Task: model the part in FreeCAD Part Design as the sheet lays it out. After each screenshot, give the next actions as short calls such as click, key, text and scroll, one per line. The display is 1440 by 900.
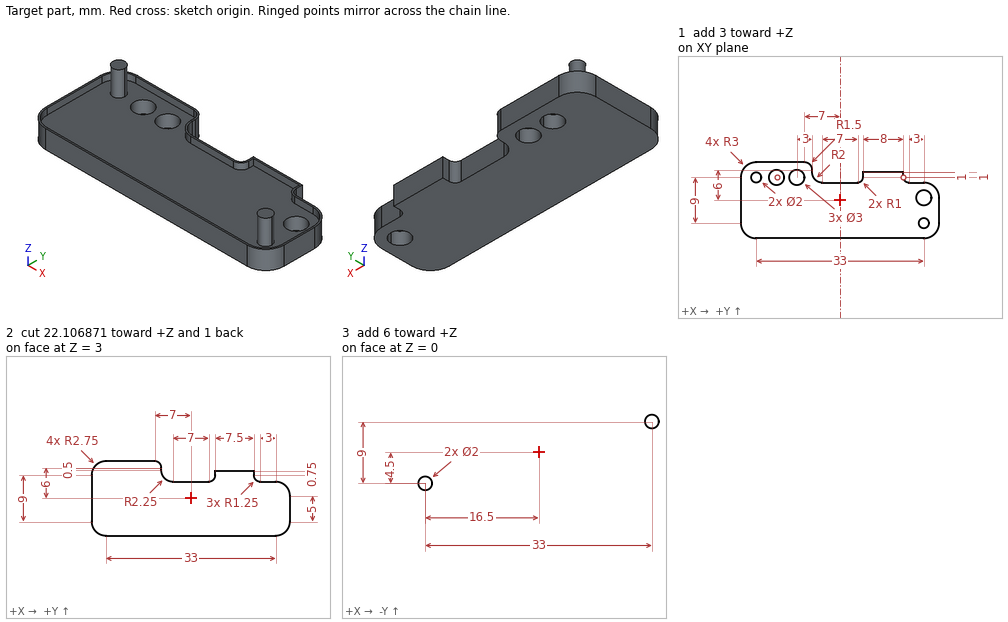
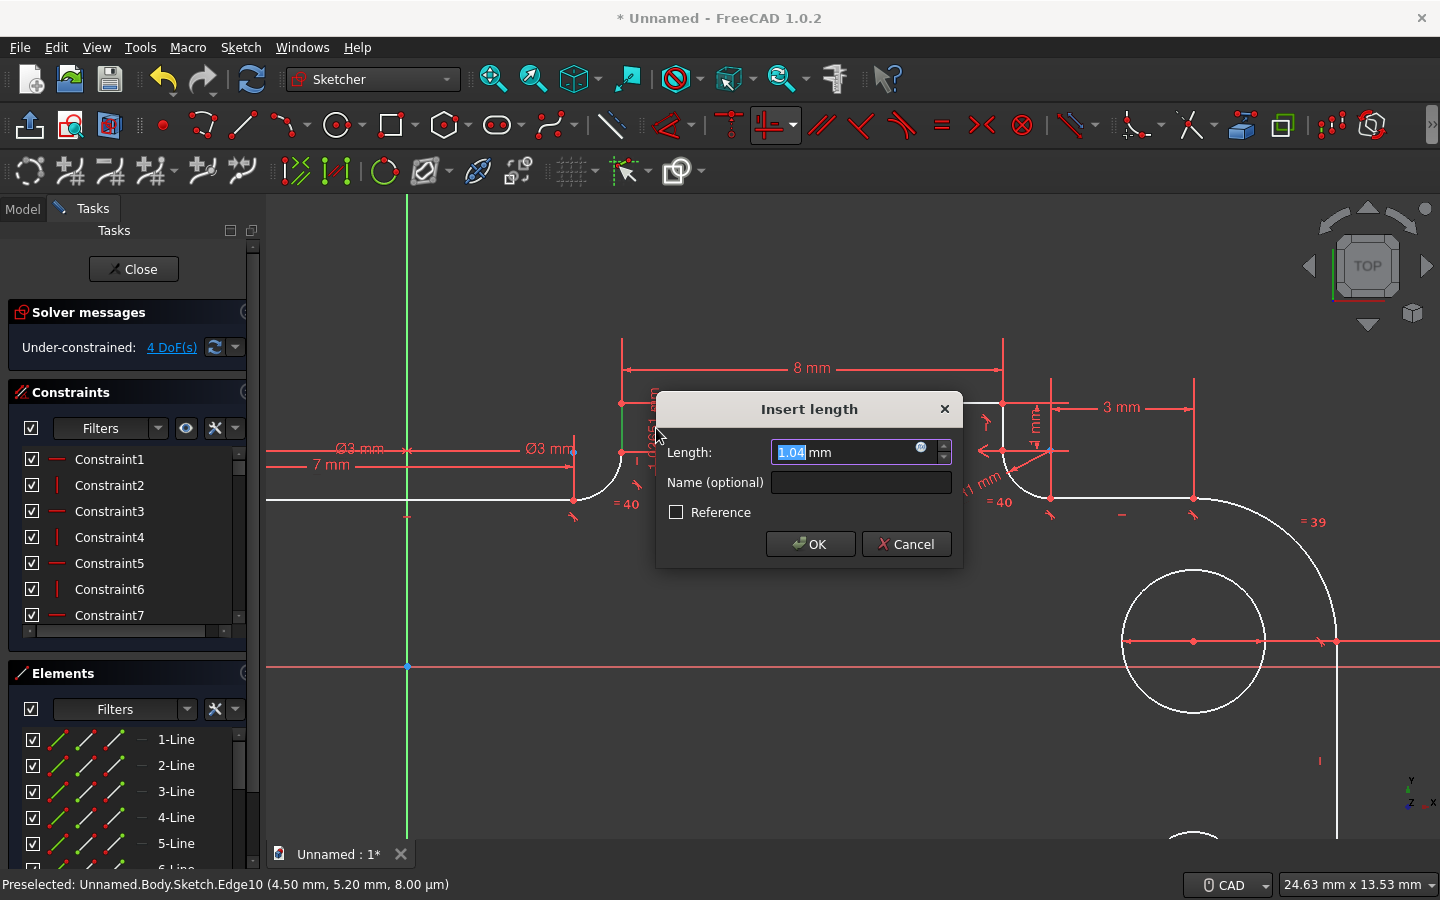
text(1)
key(Return)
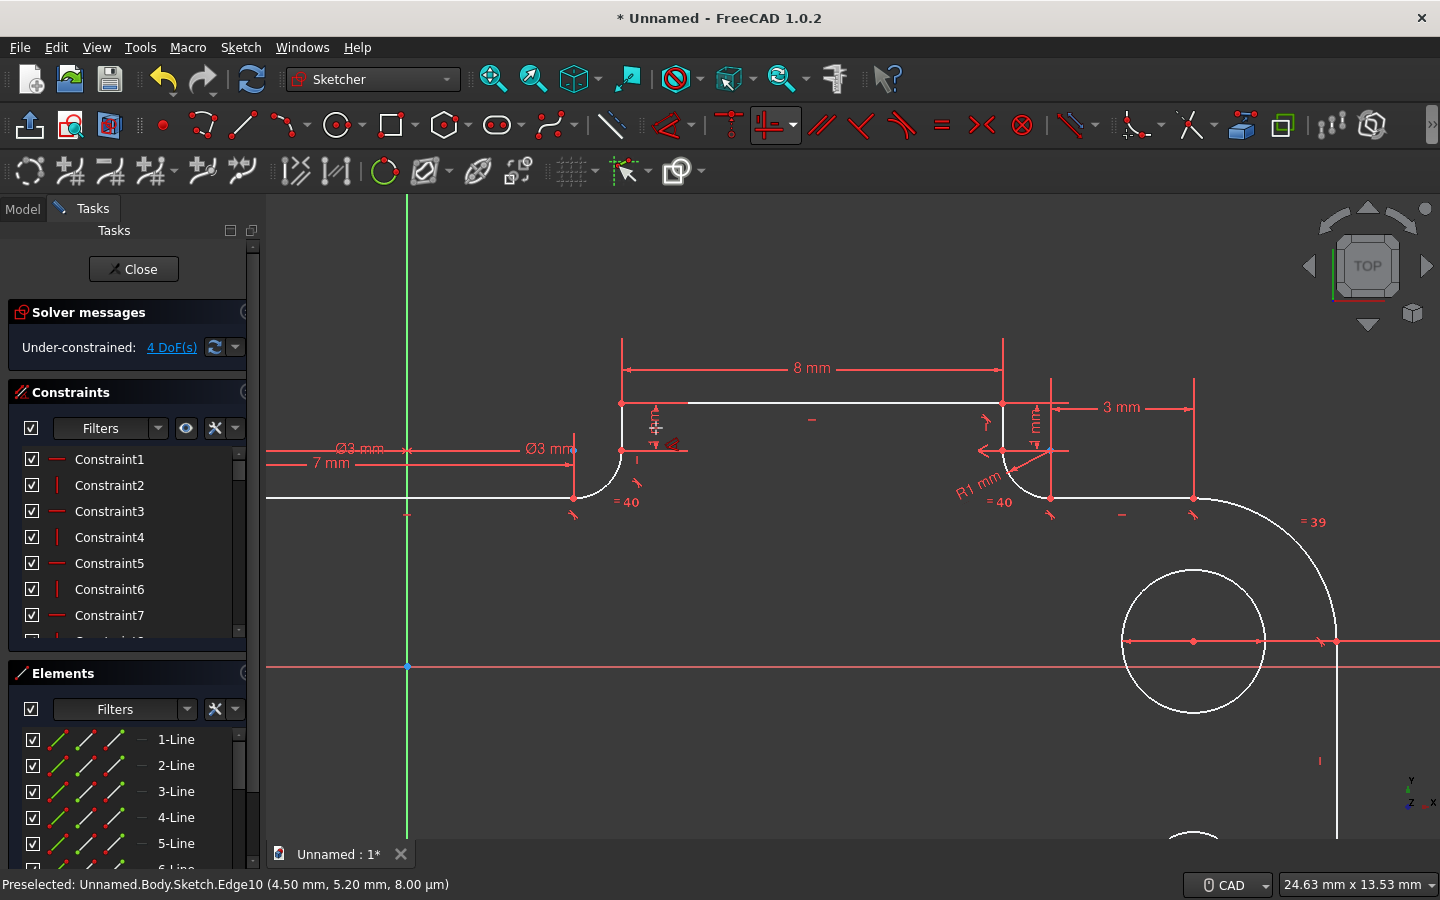
scroll(1004, 429, down, 5)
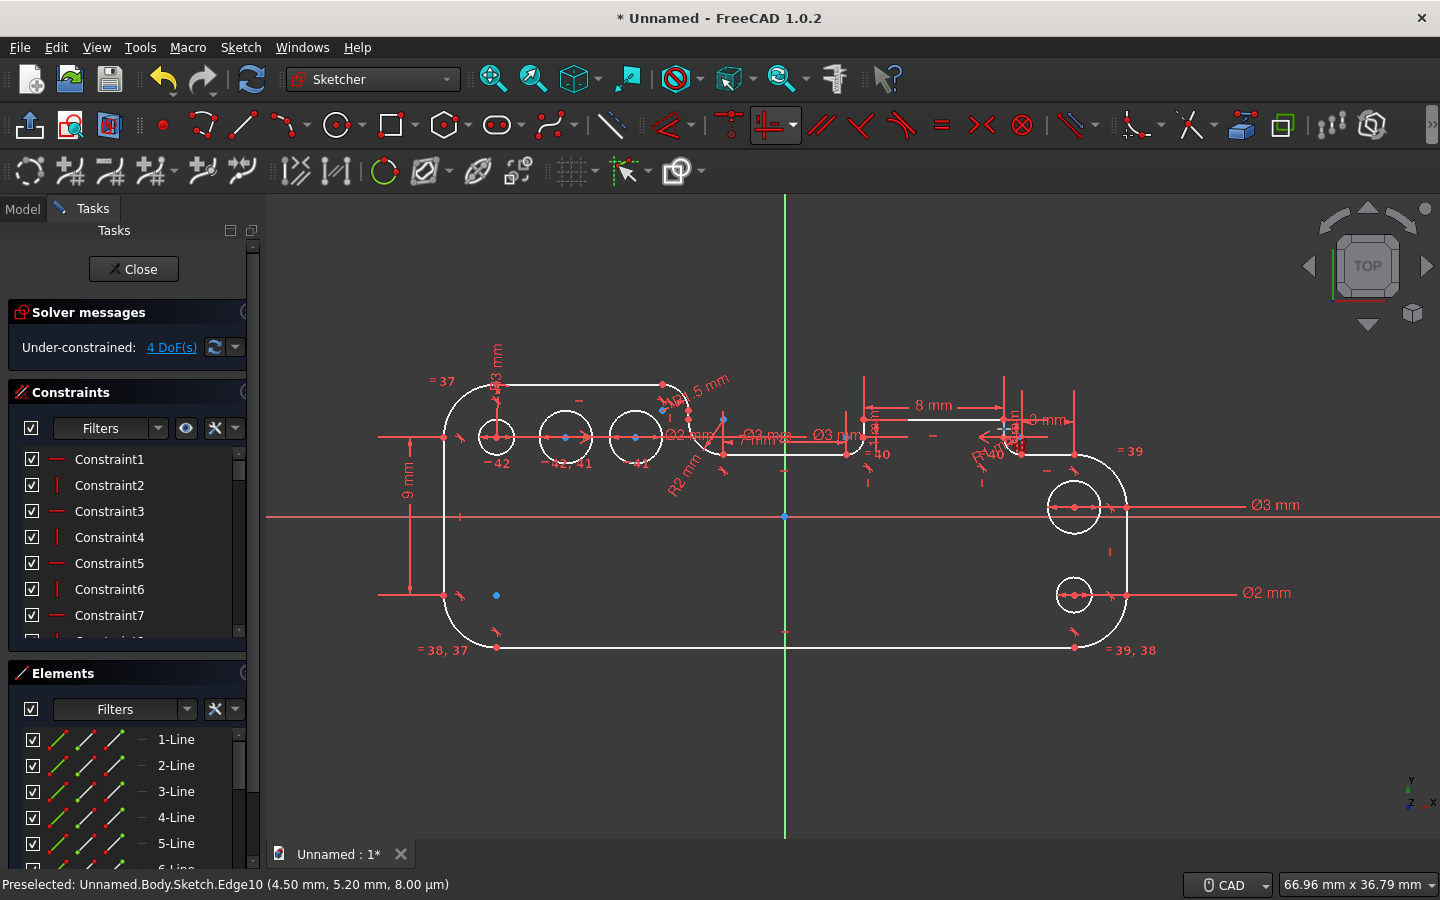
click(670, 648)
click(653, 682)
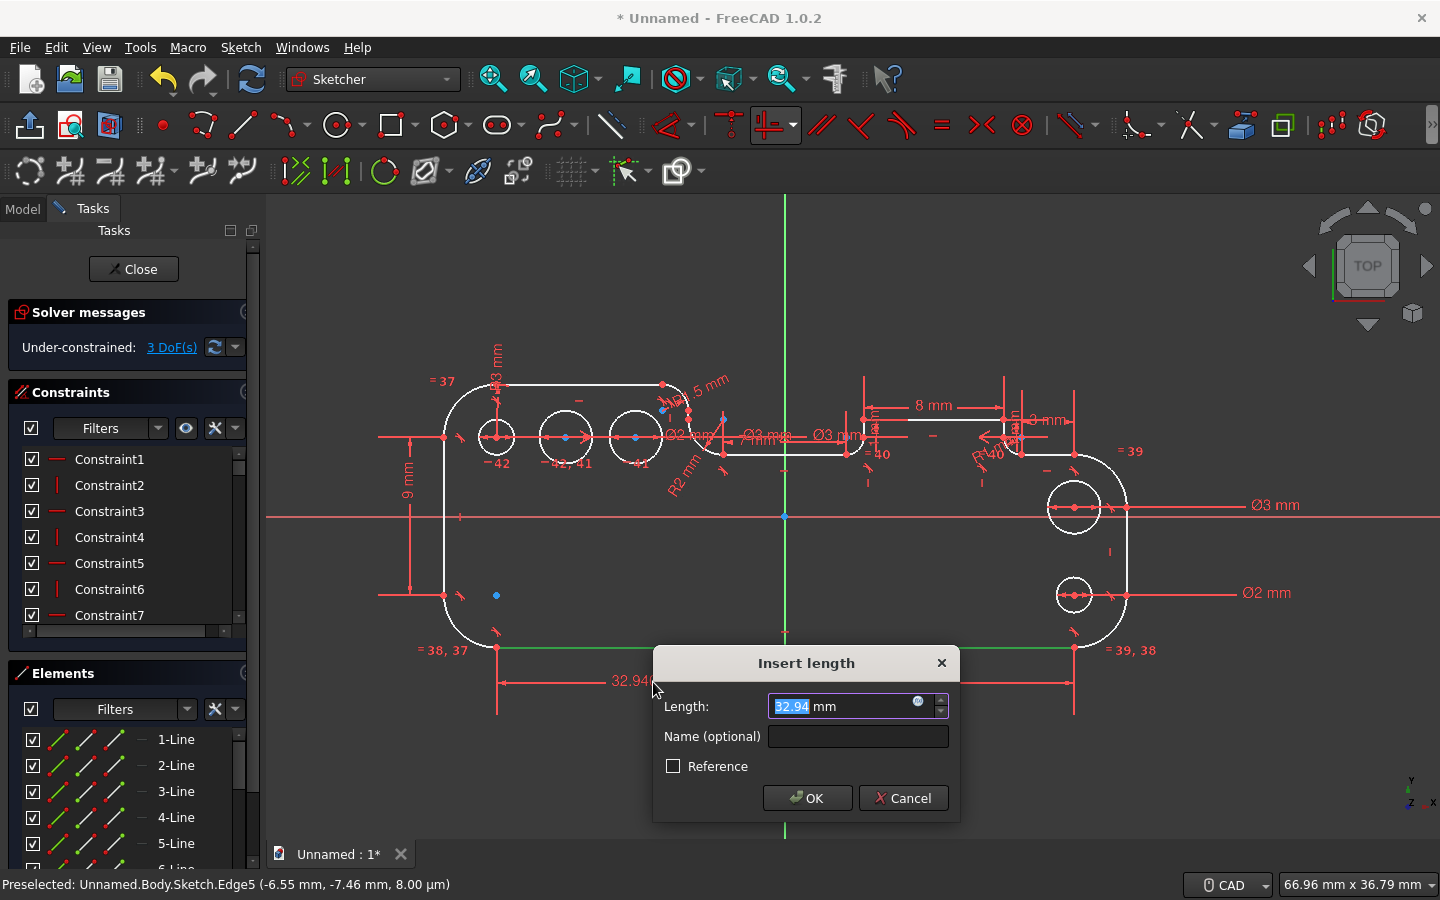
text(33)
key(Return)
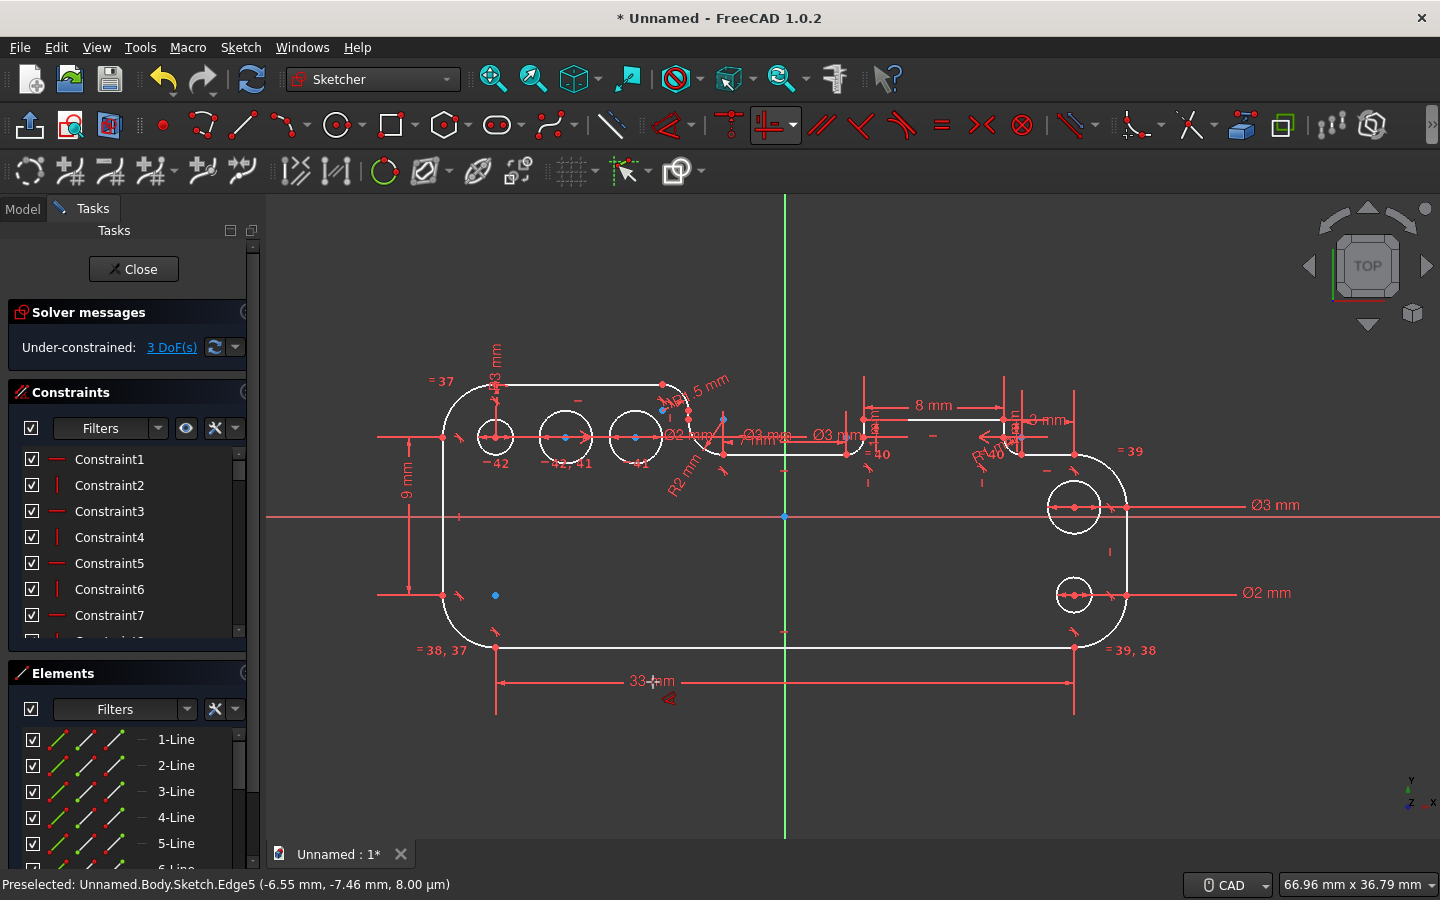
scroll(688, 411, up, 2)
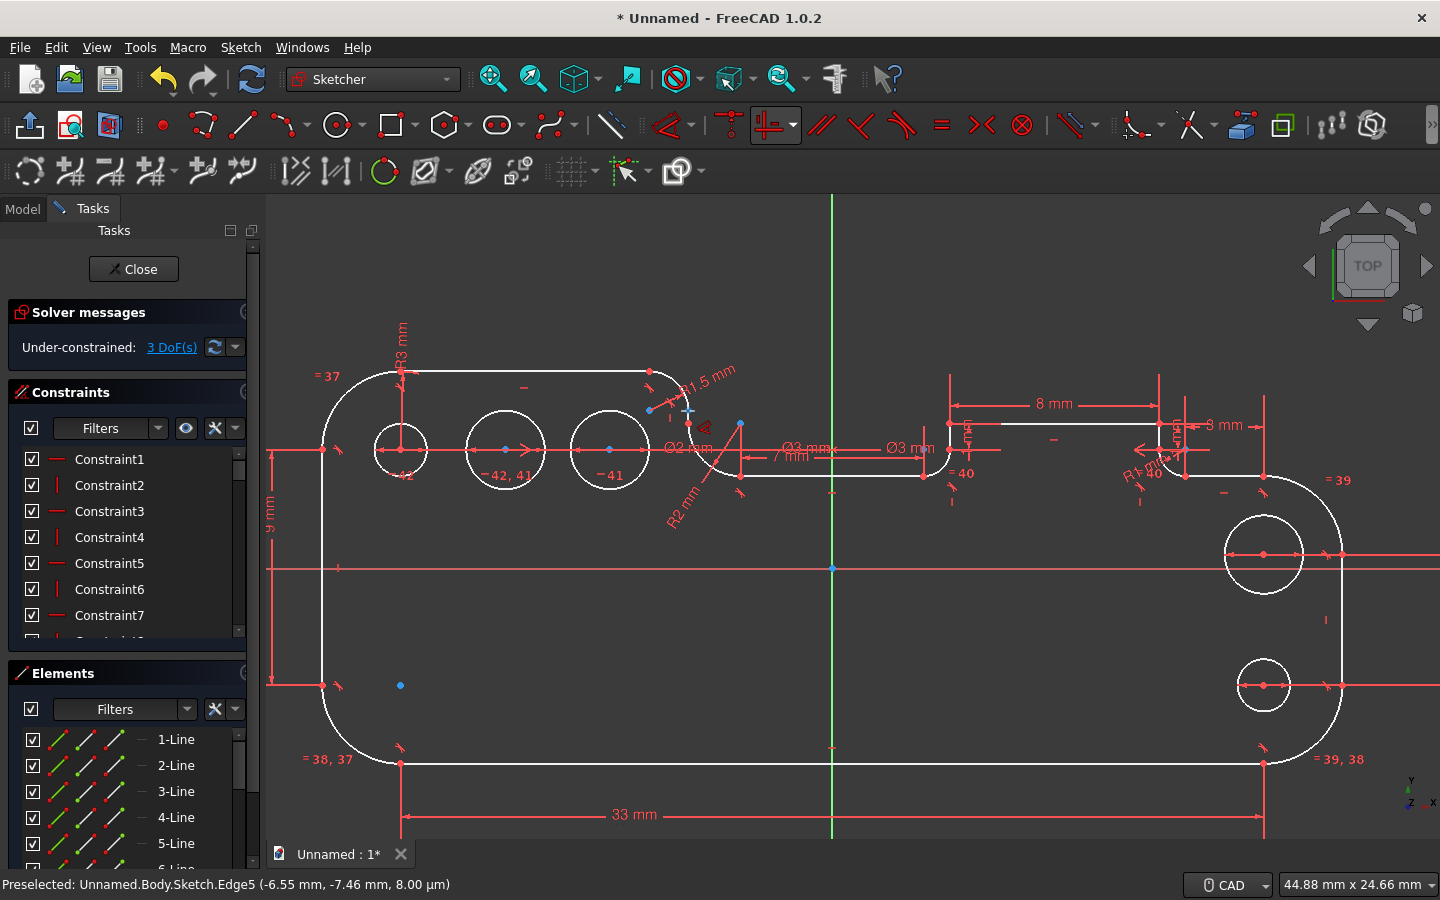
click(688, 411)
click(654, 545)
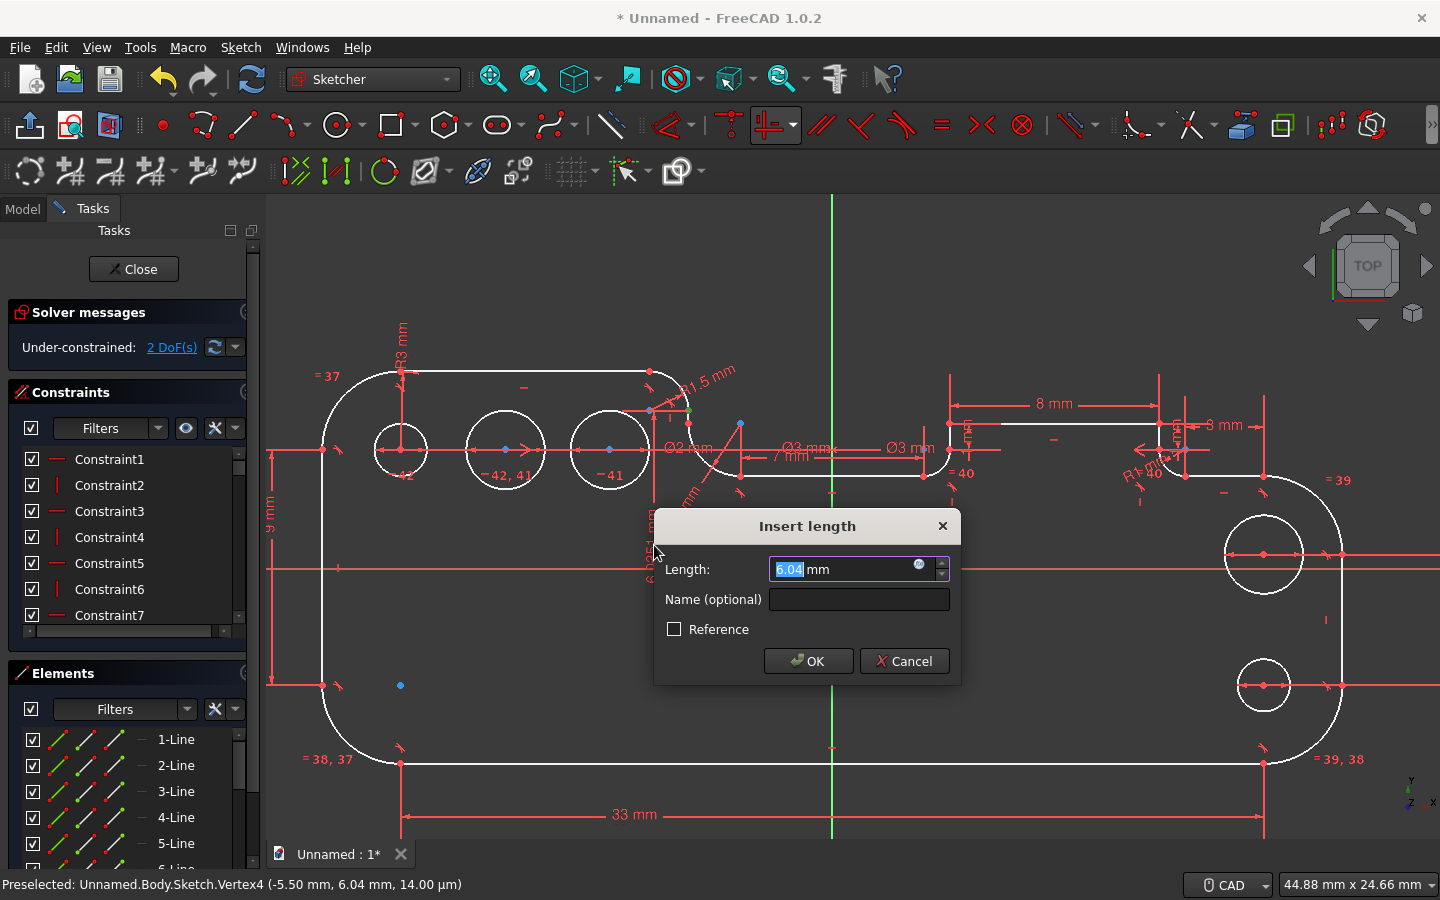
text(6)
key(Return)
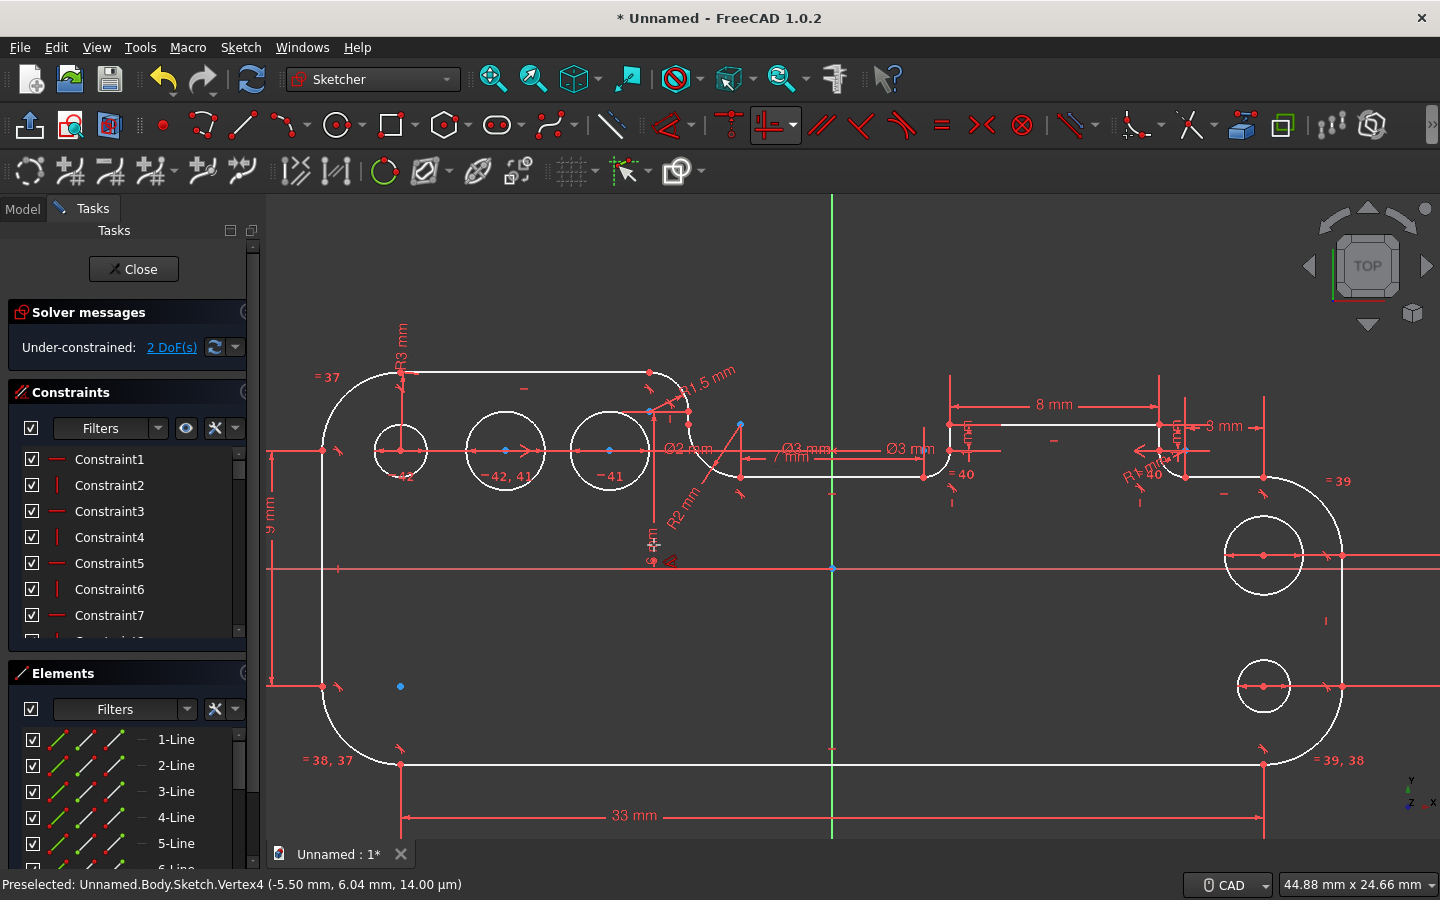
click(649, 372)
click(741, 338)